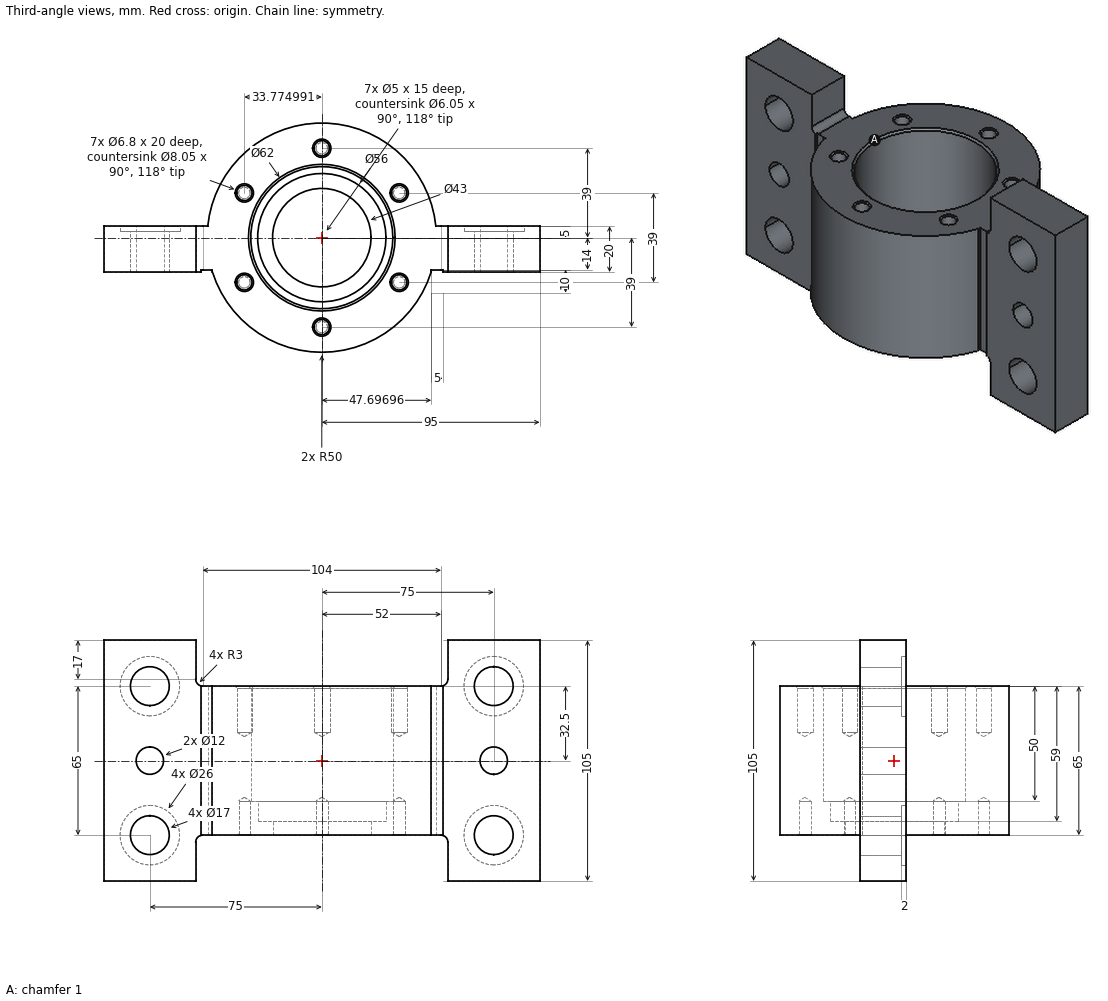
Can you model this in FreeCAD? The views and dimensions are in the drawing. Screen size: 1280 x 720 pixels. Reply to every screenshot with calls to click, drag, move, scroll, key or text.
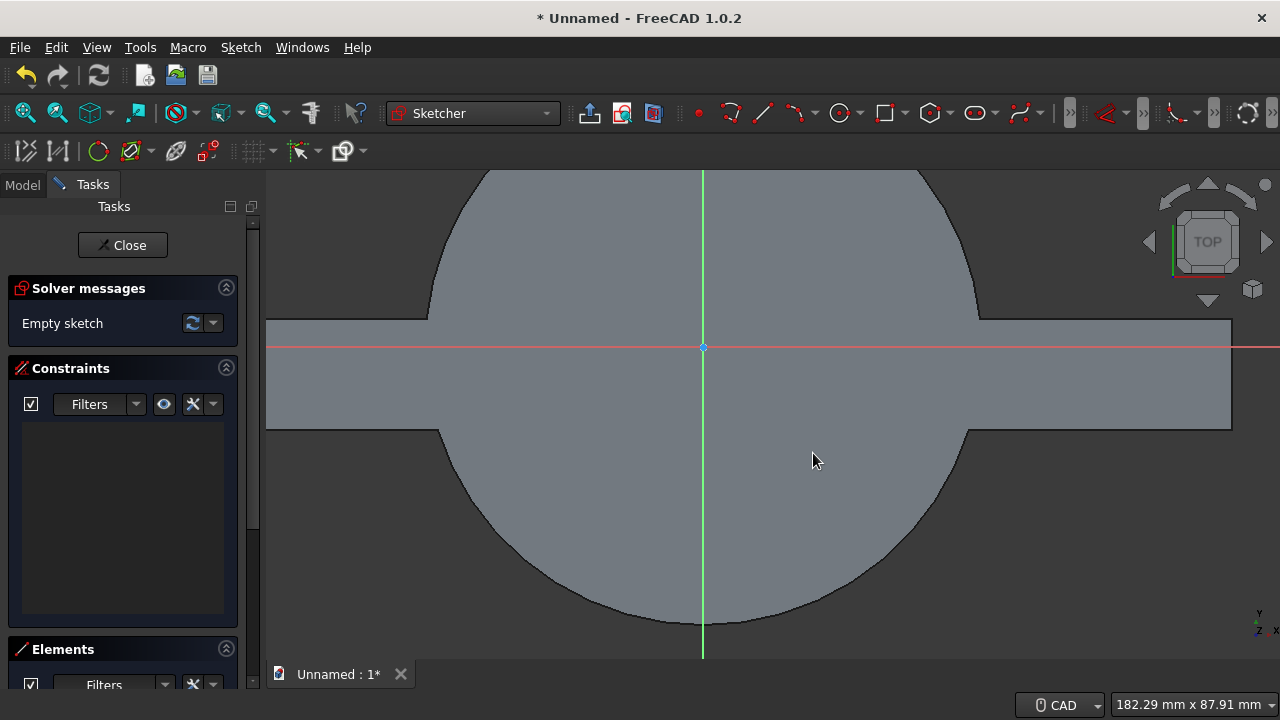
click(886, 114)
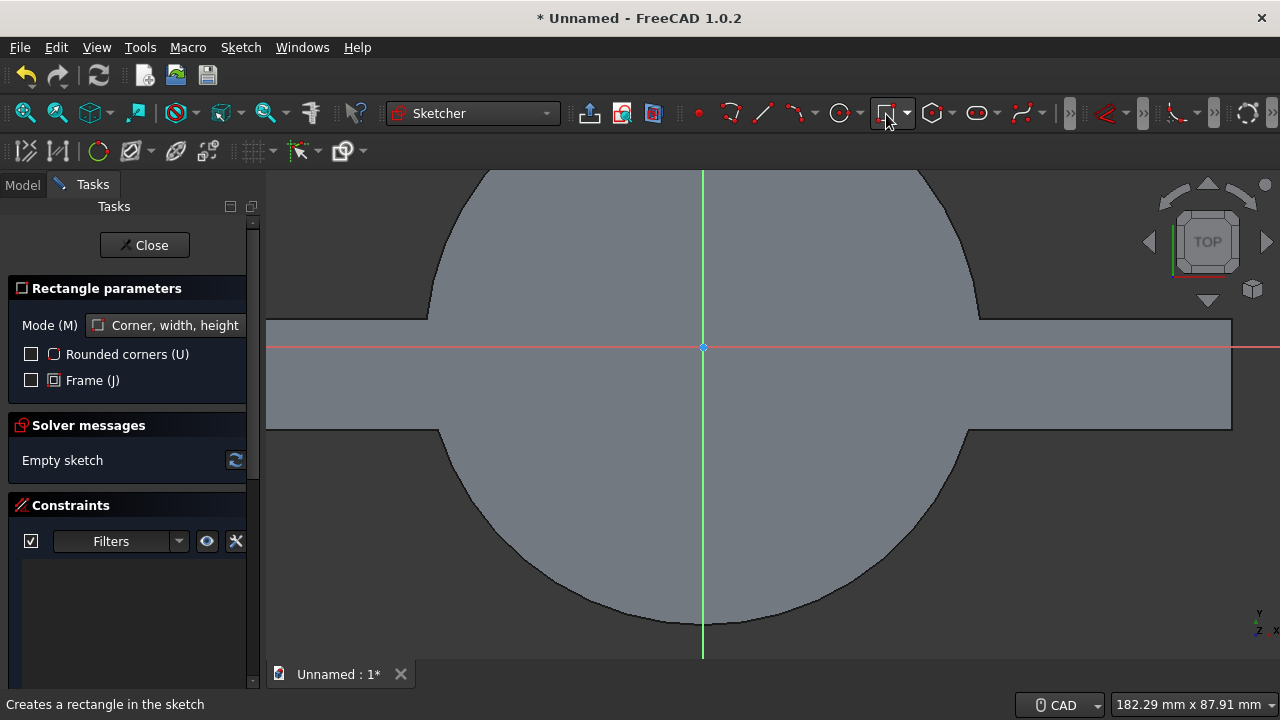
click(969, 425)
click(996, 481)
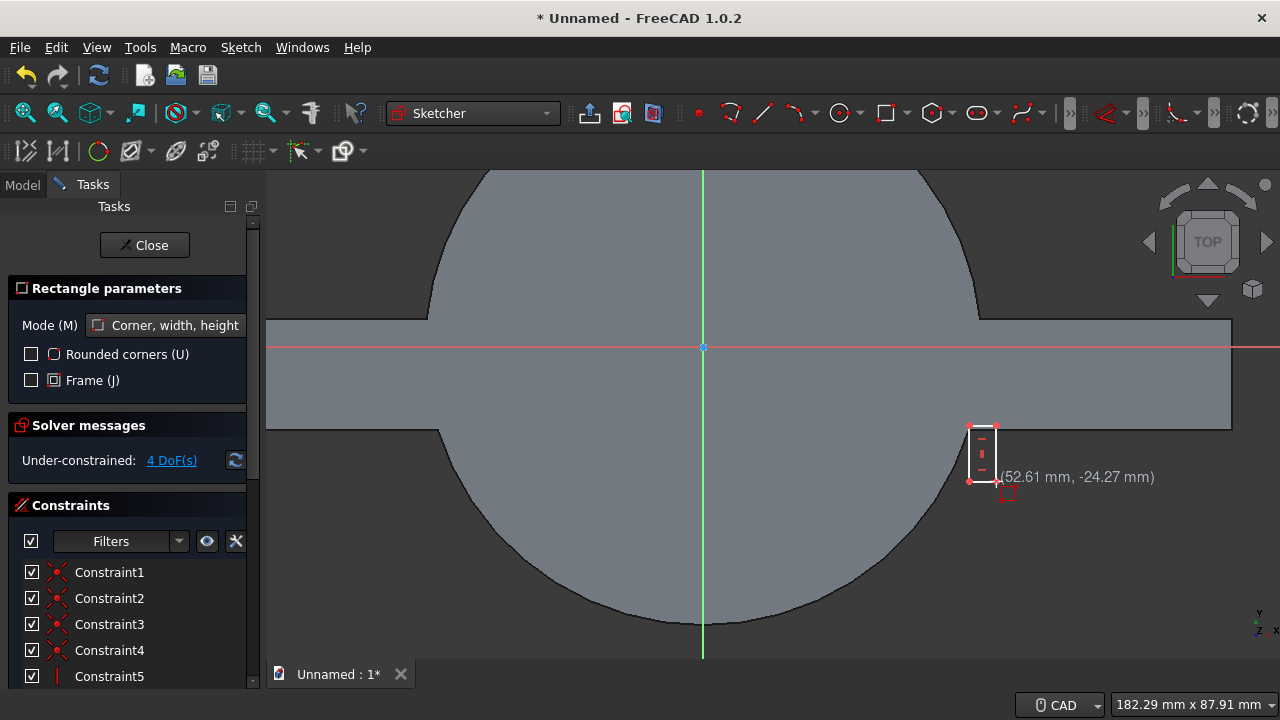
click(410, 425)
click(438, 481)
key(Escape)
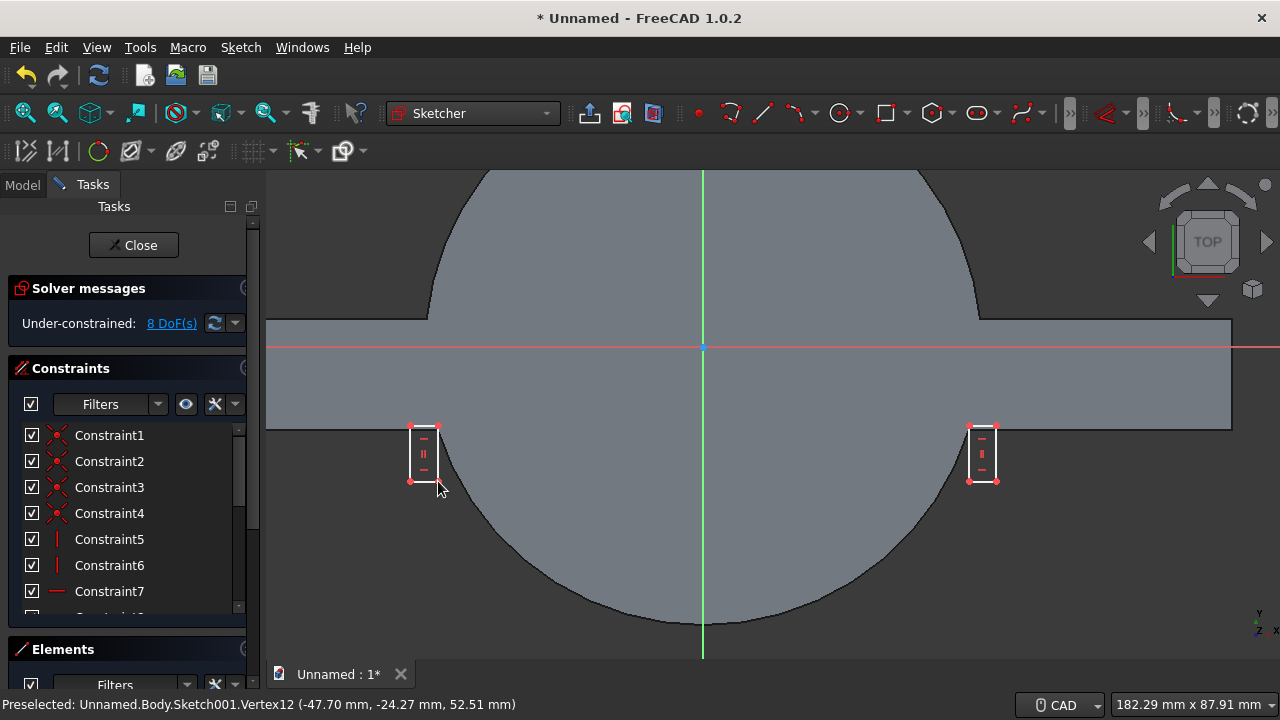
click(996, 426)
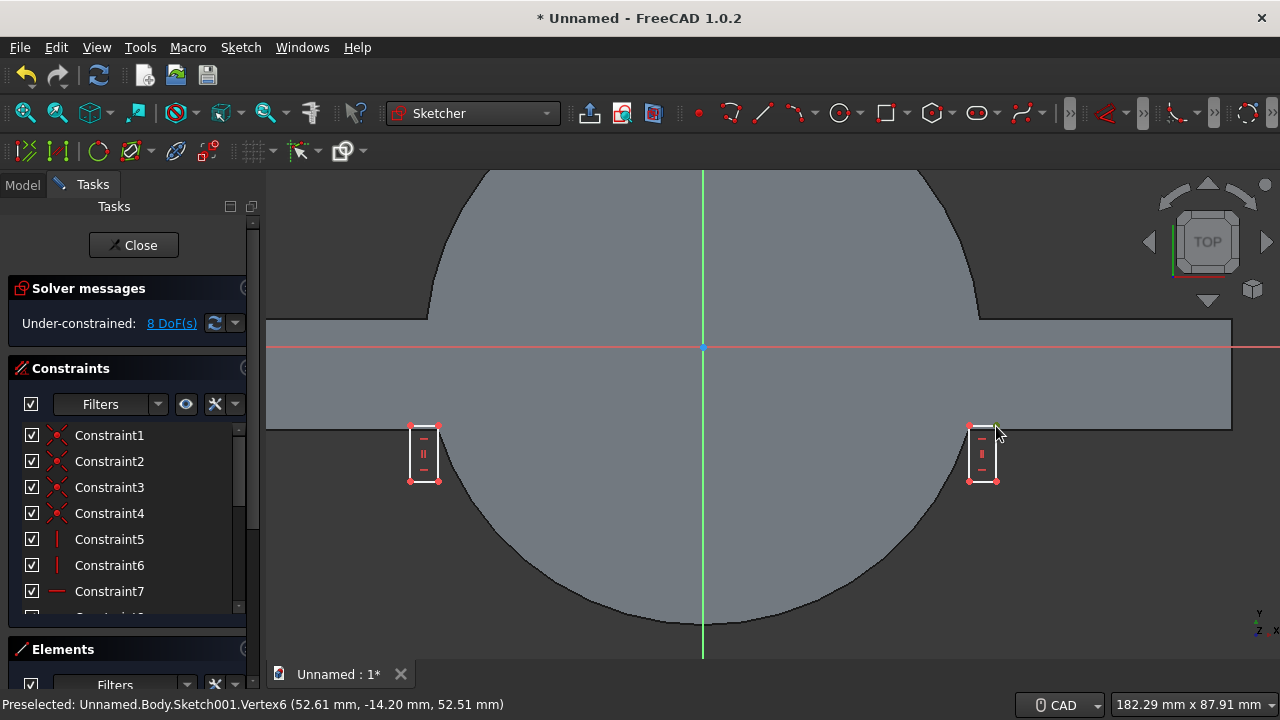
click(410, 426)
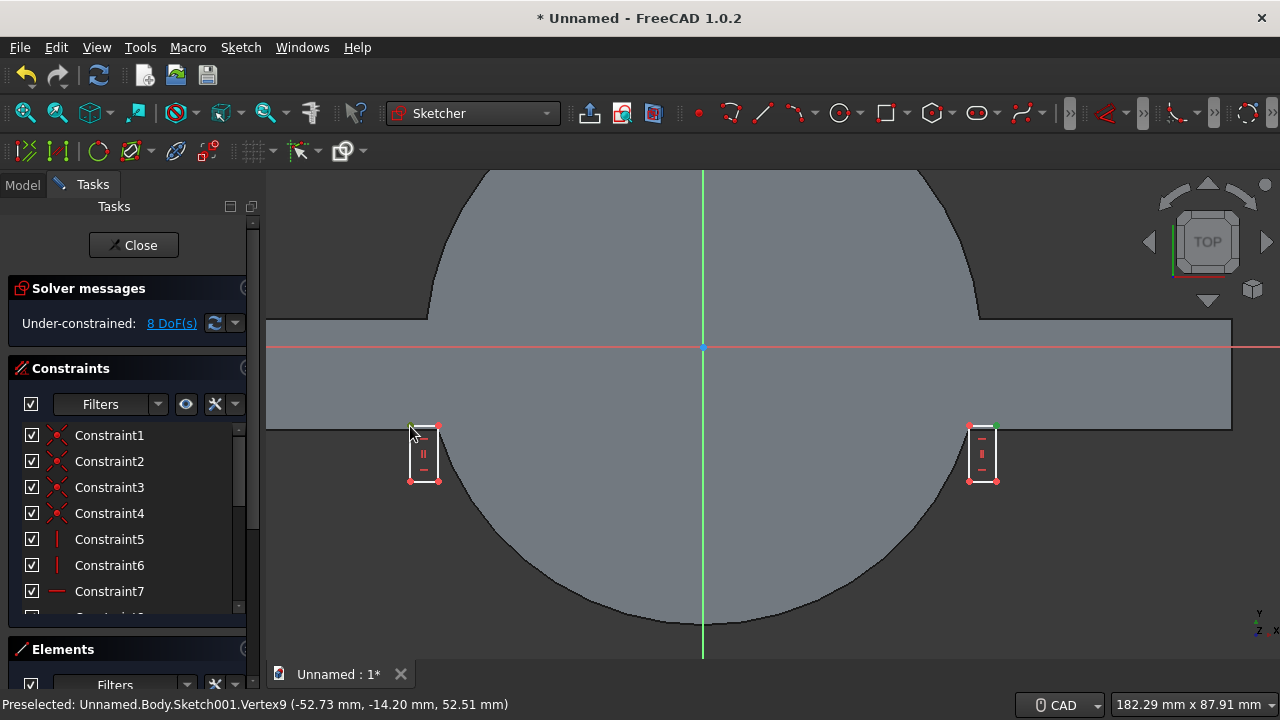
click(703, 600)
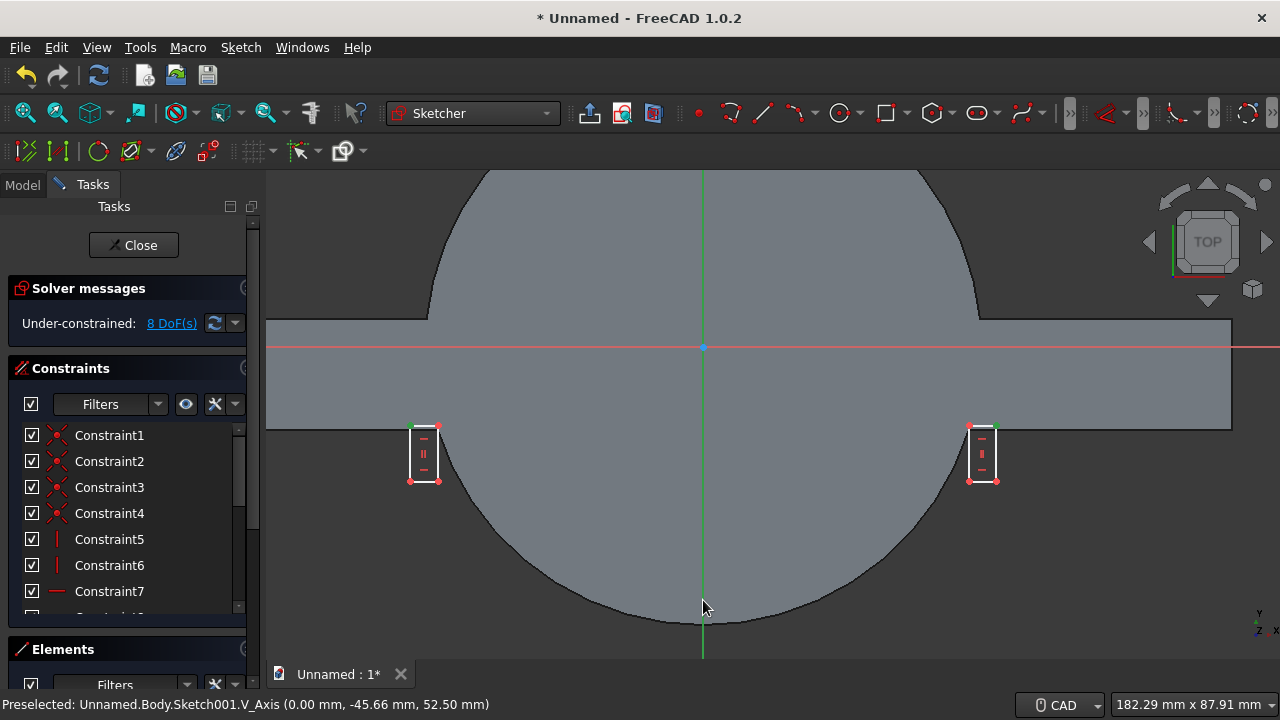
key(s)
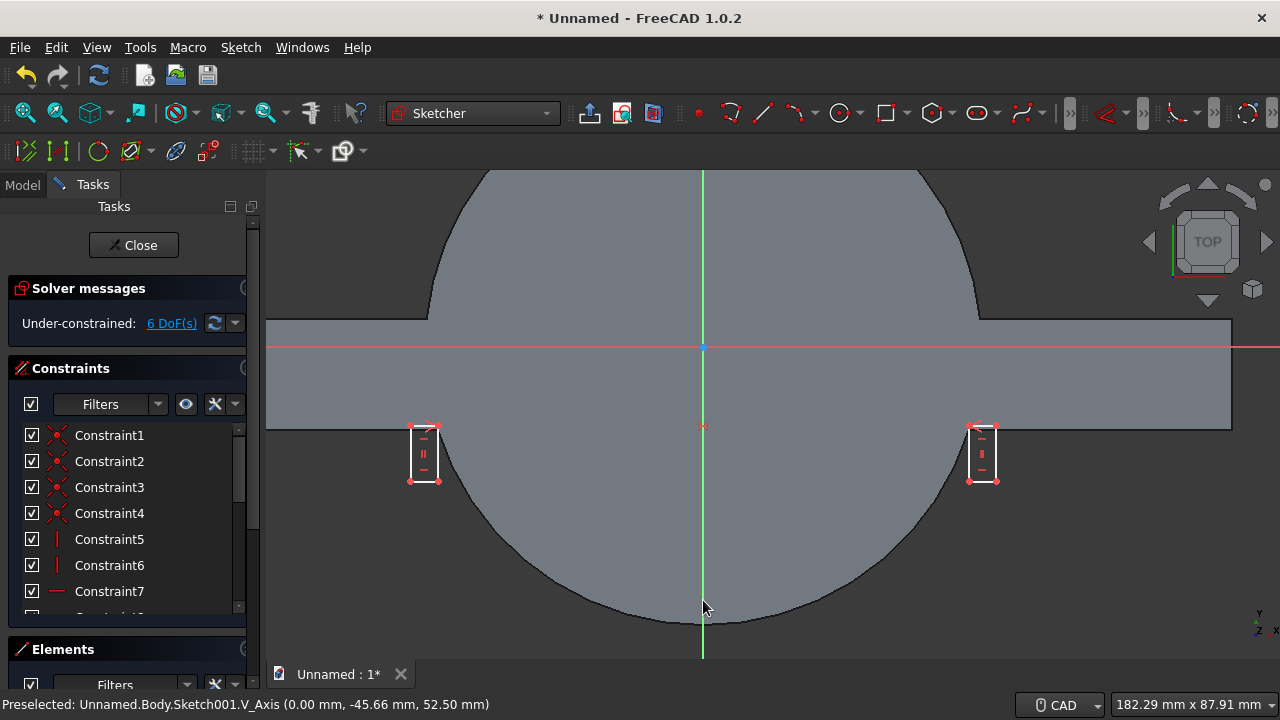
click(969, 482)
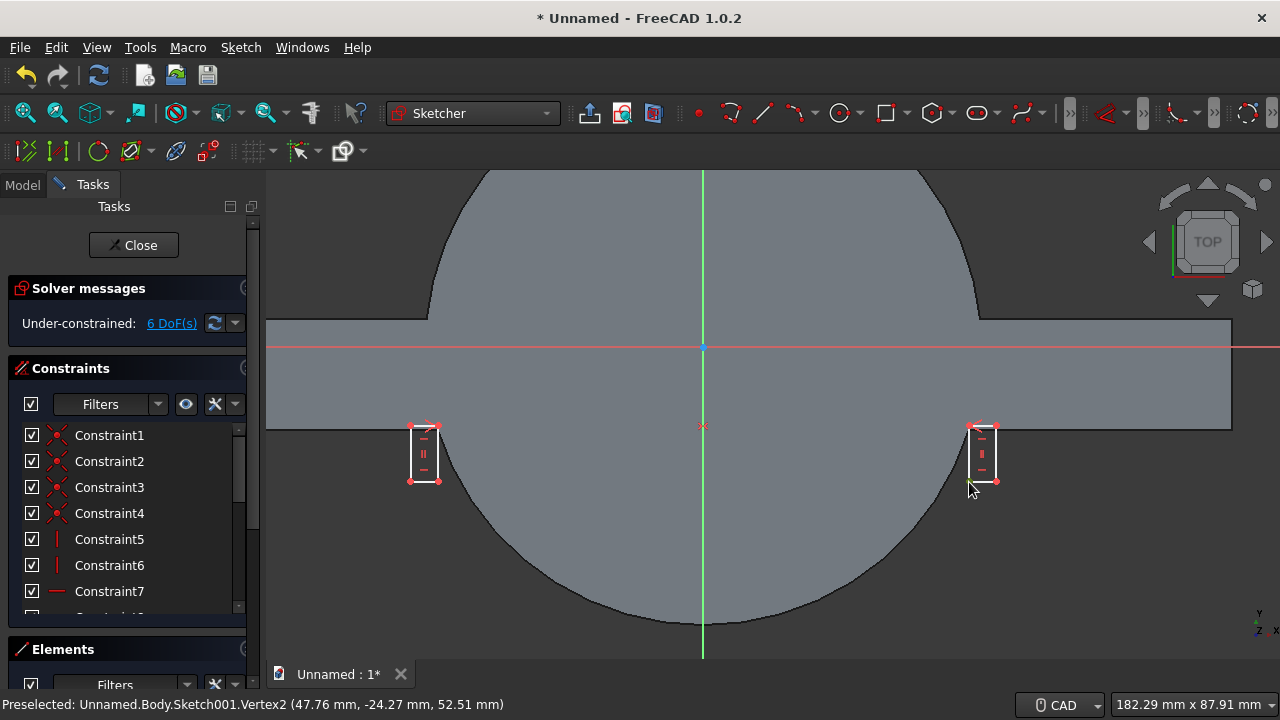
click(438, 482)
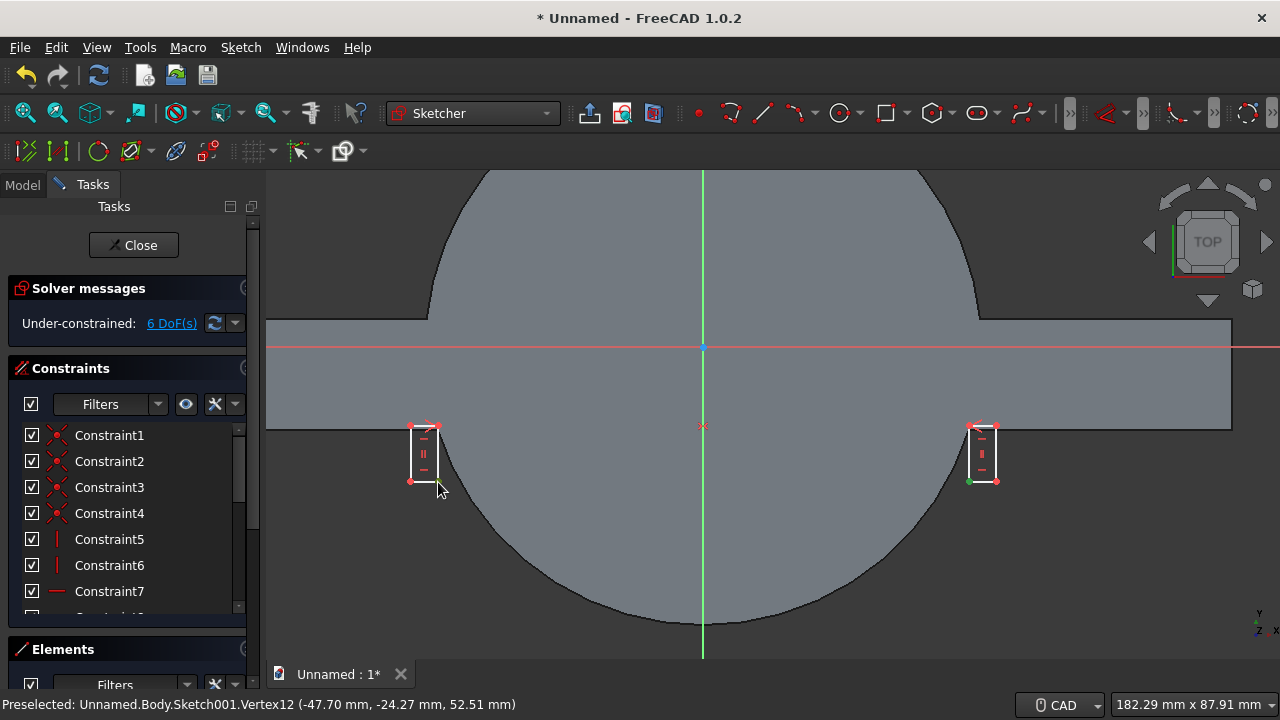
click(703, 600)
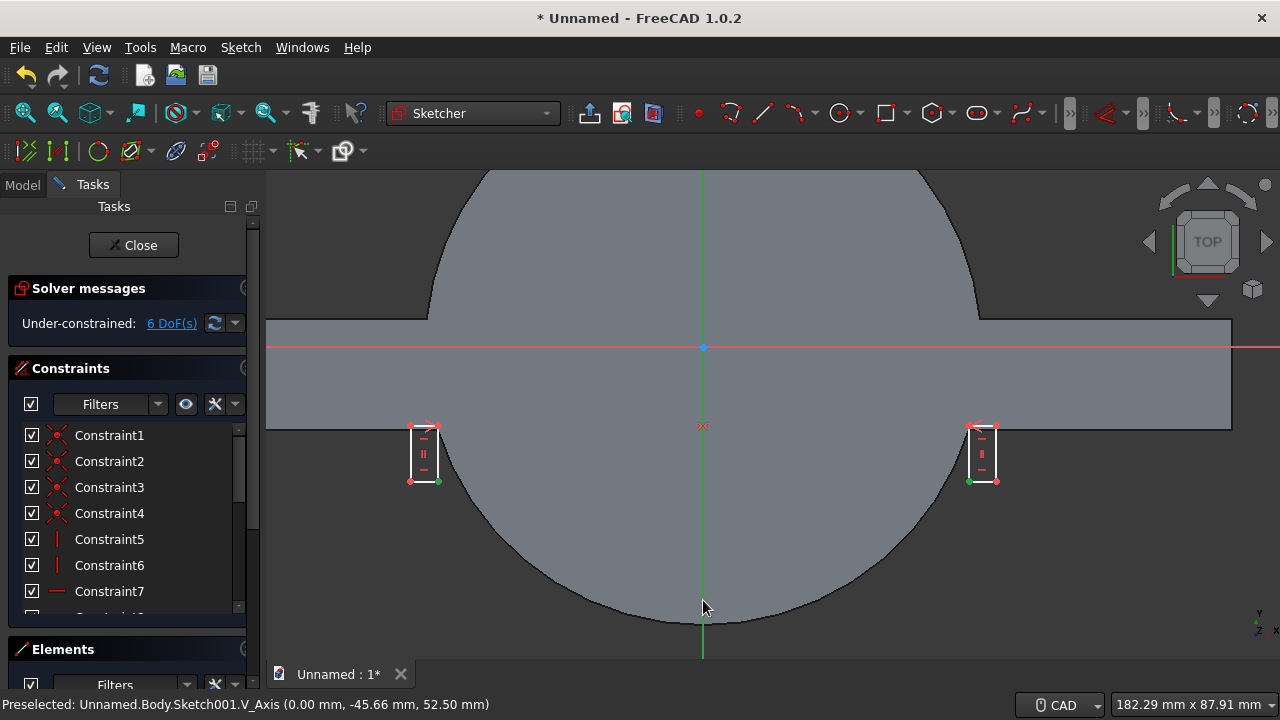
key(s)